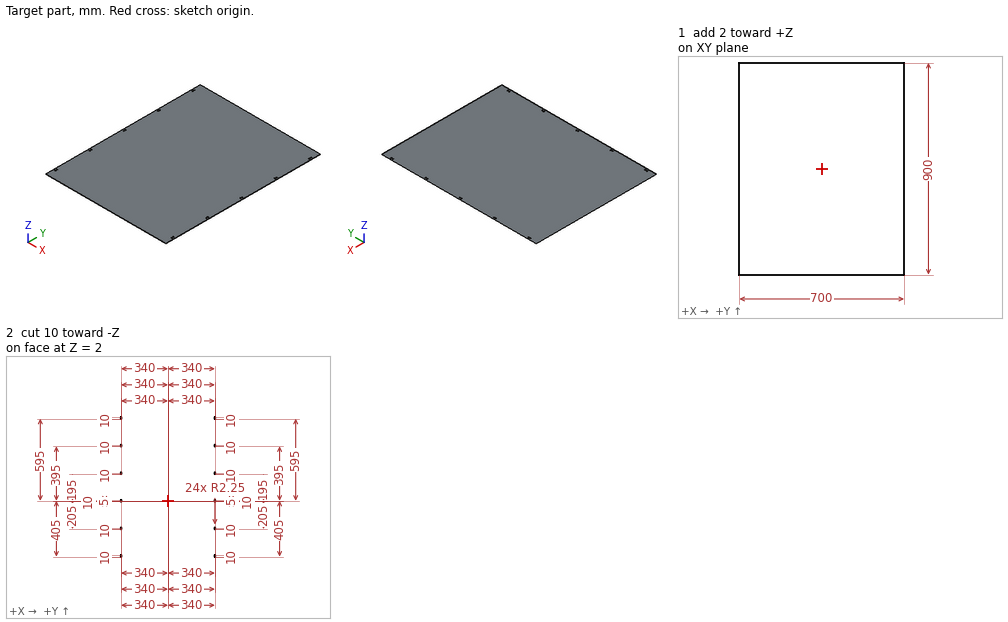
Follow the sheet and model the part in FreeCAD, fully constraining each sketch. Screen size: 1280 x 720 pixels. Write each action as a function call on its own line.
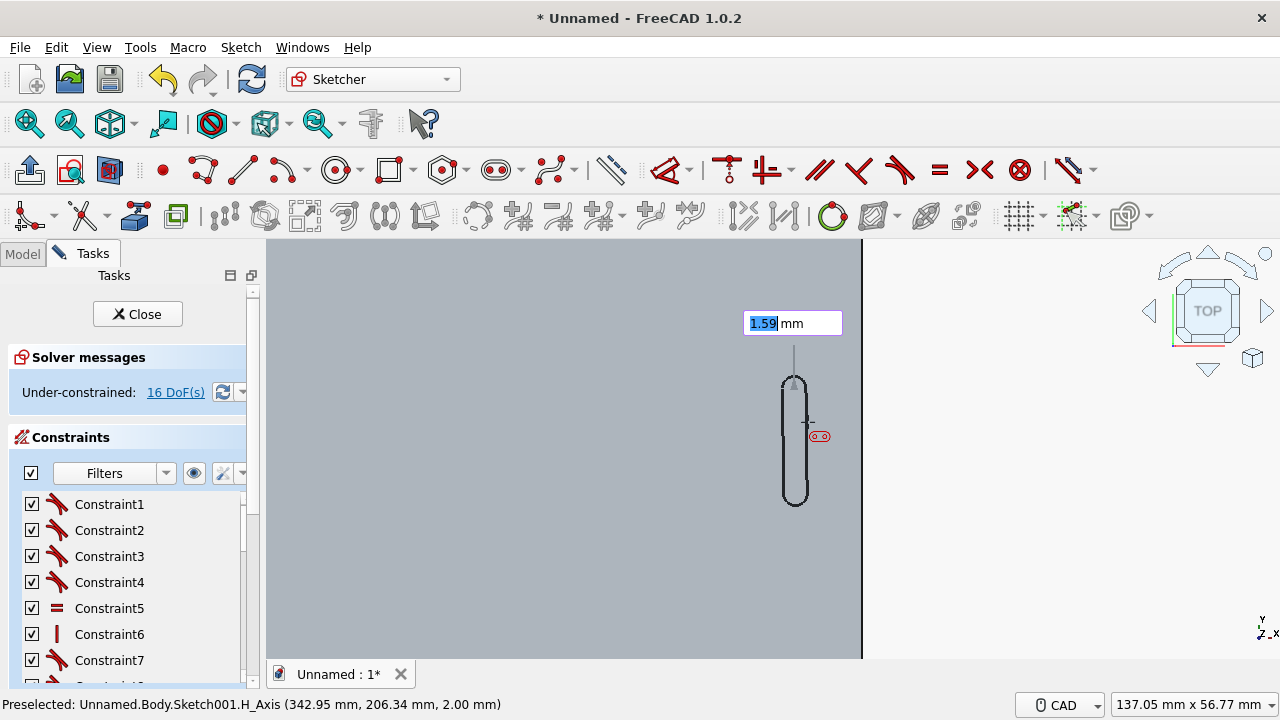
click(804, 422)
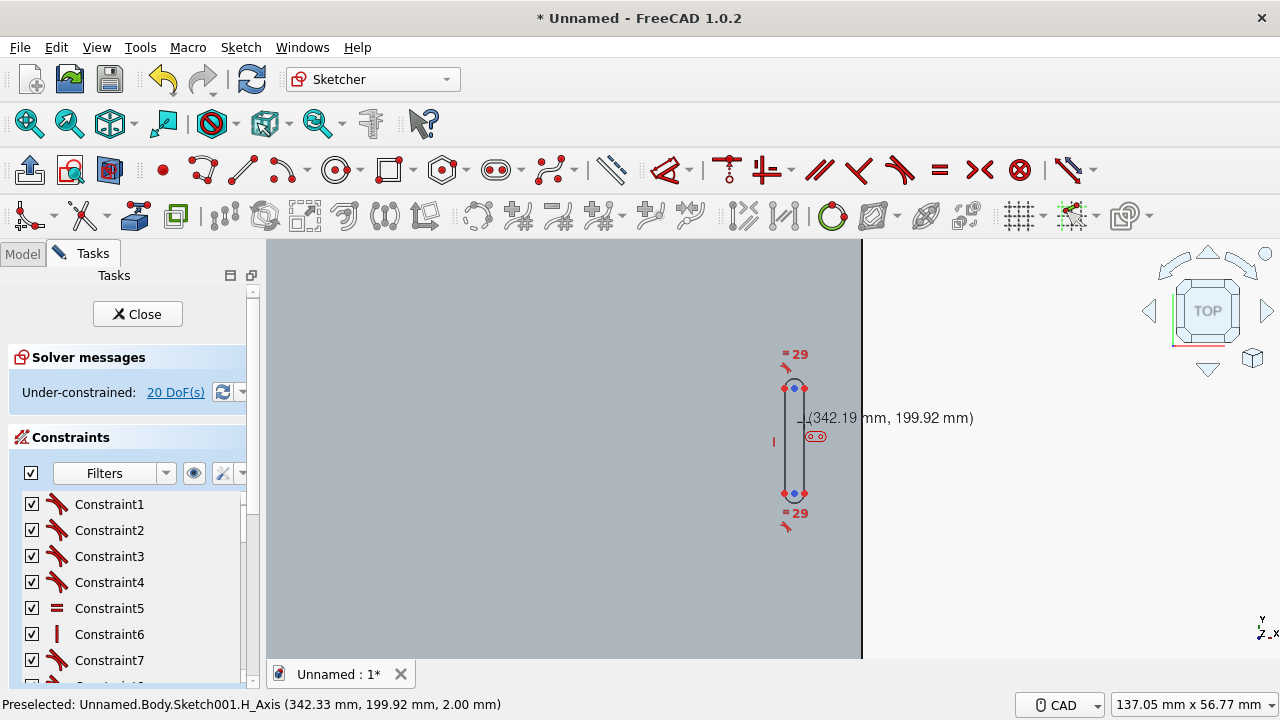
scroll(808, 419, down, 16)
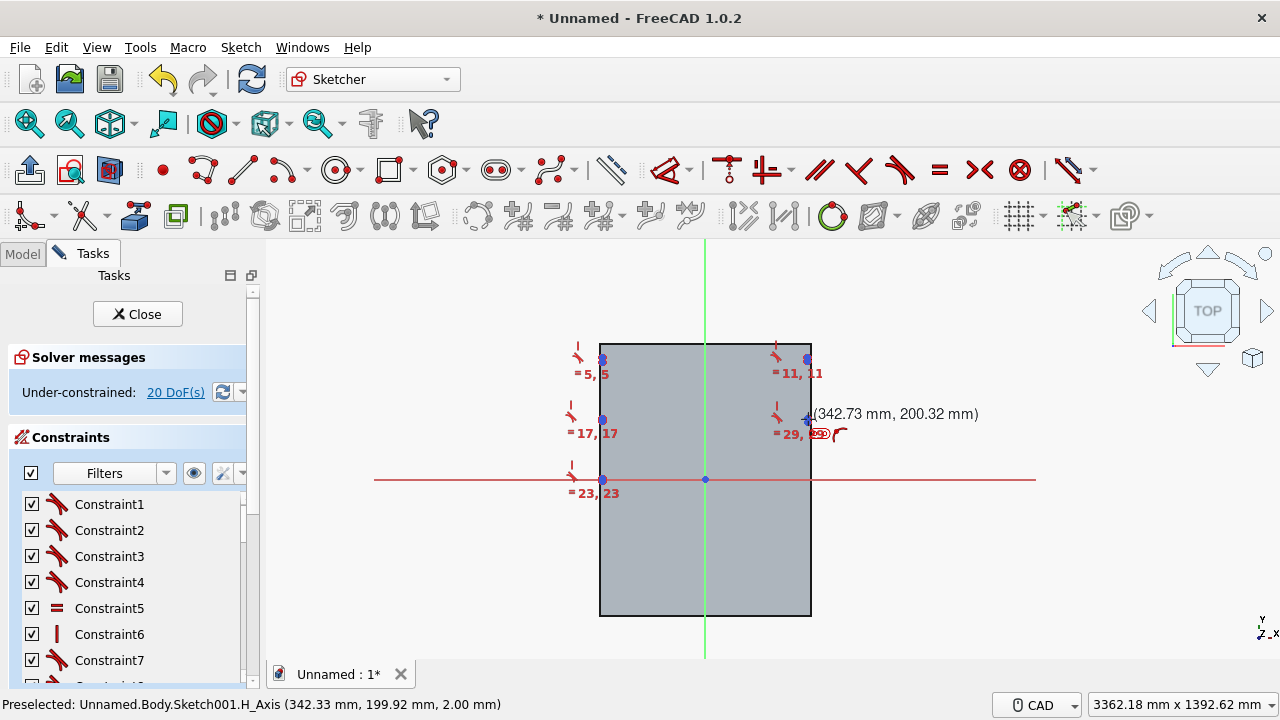
scroll(808, 481, up, 18)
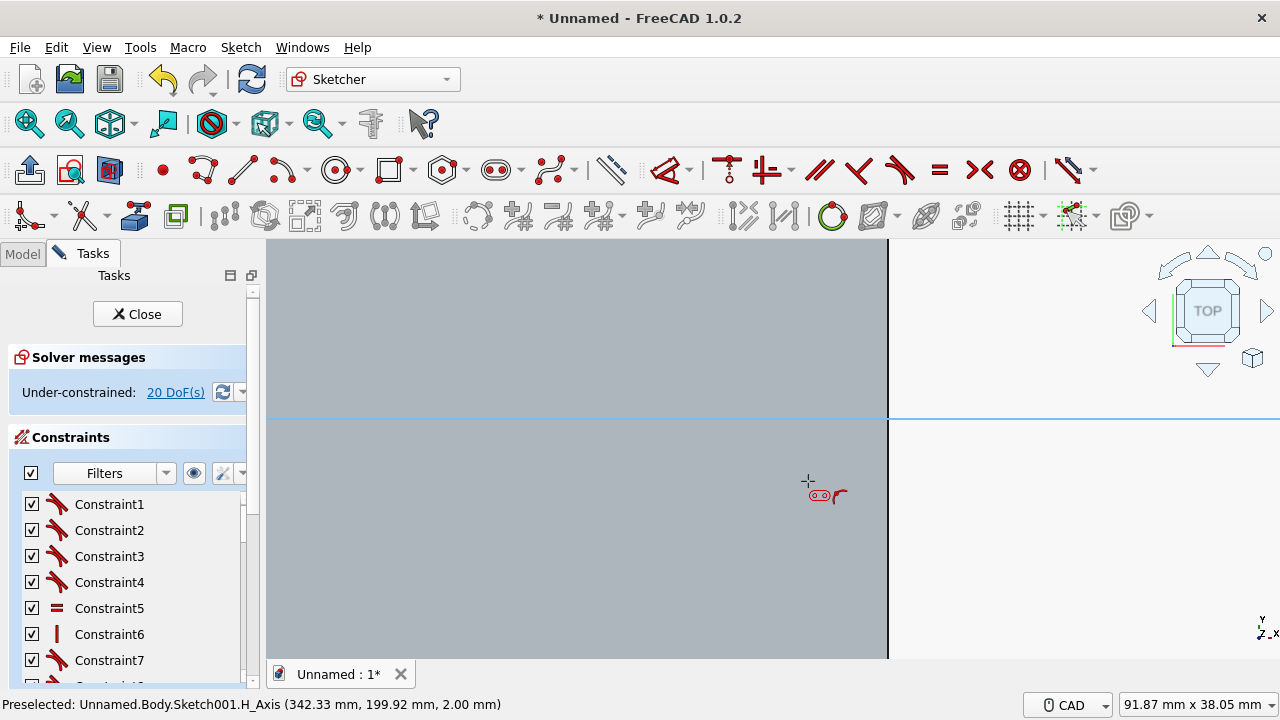
scroll(808, 481, down, 18)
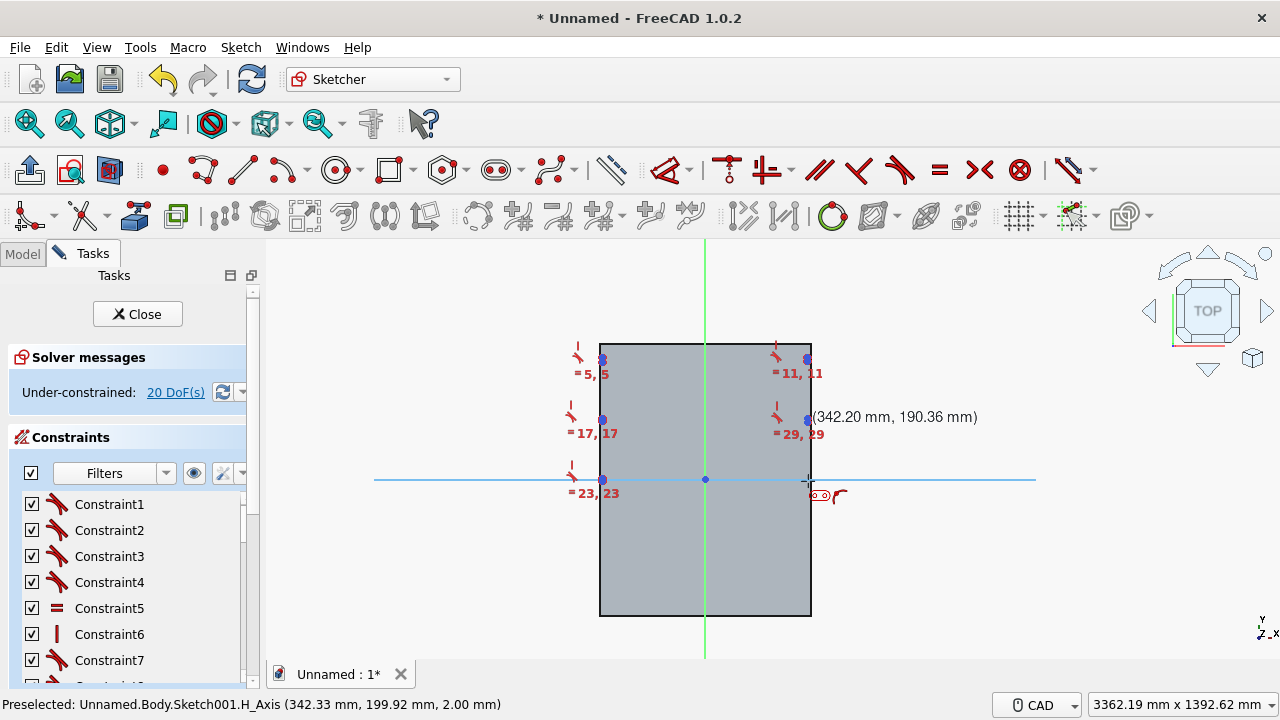
scroll(808, 481, up, 12)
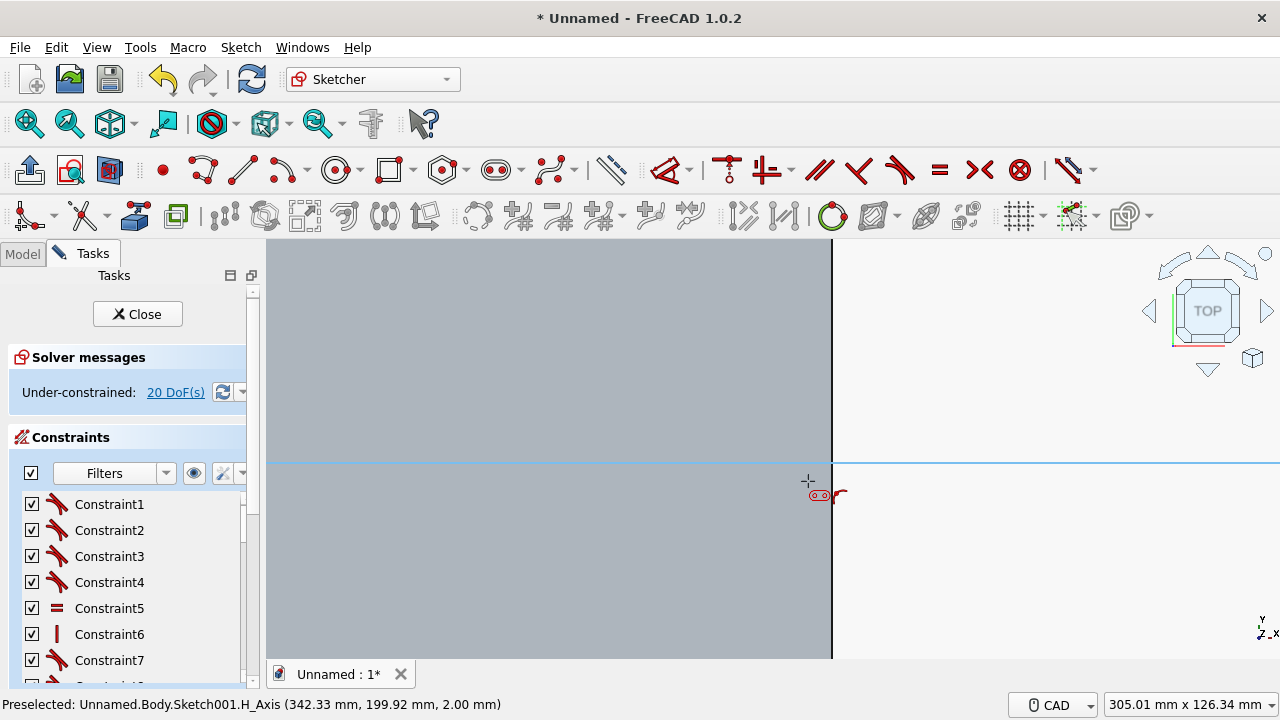
click(799, 479)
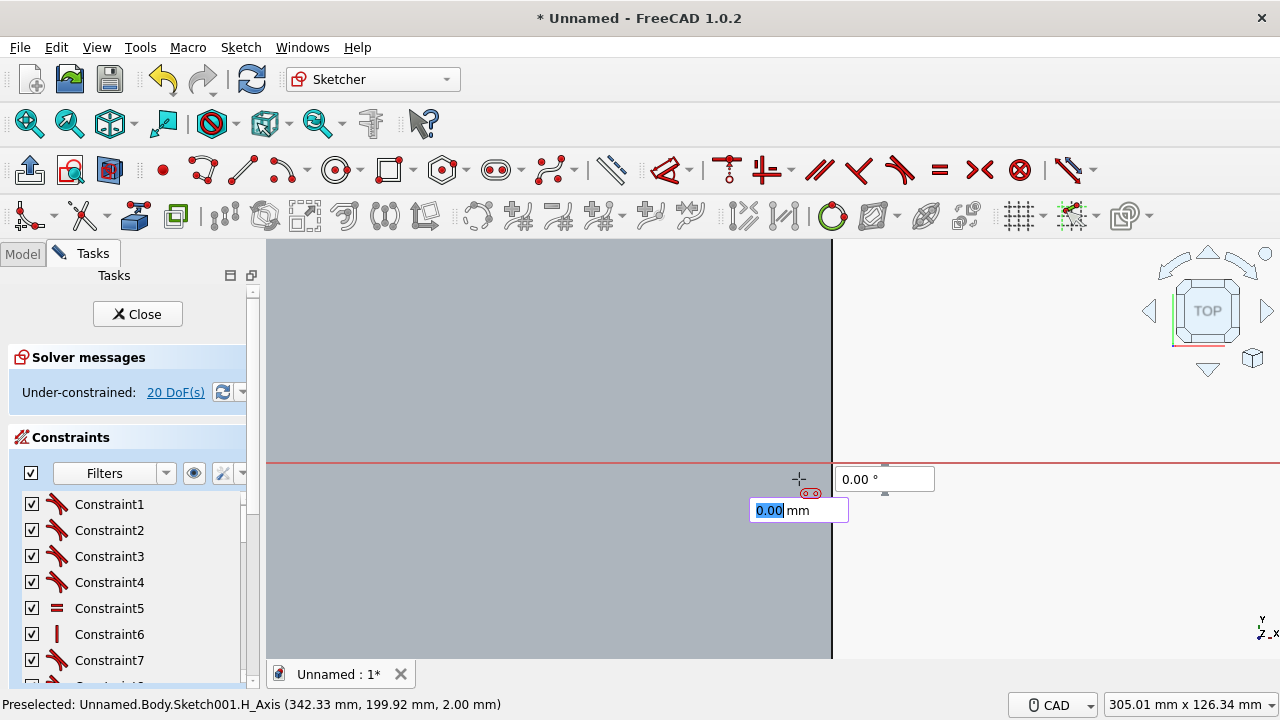
click(799, 446)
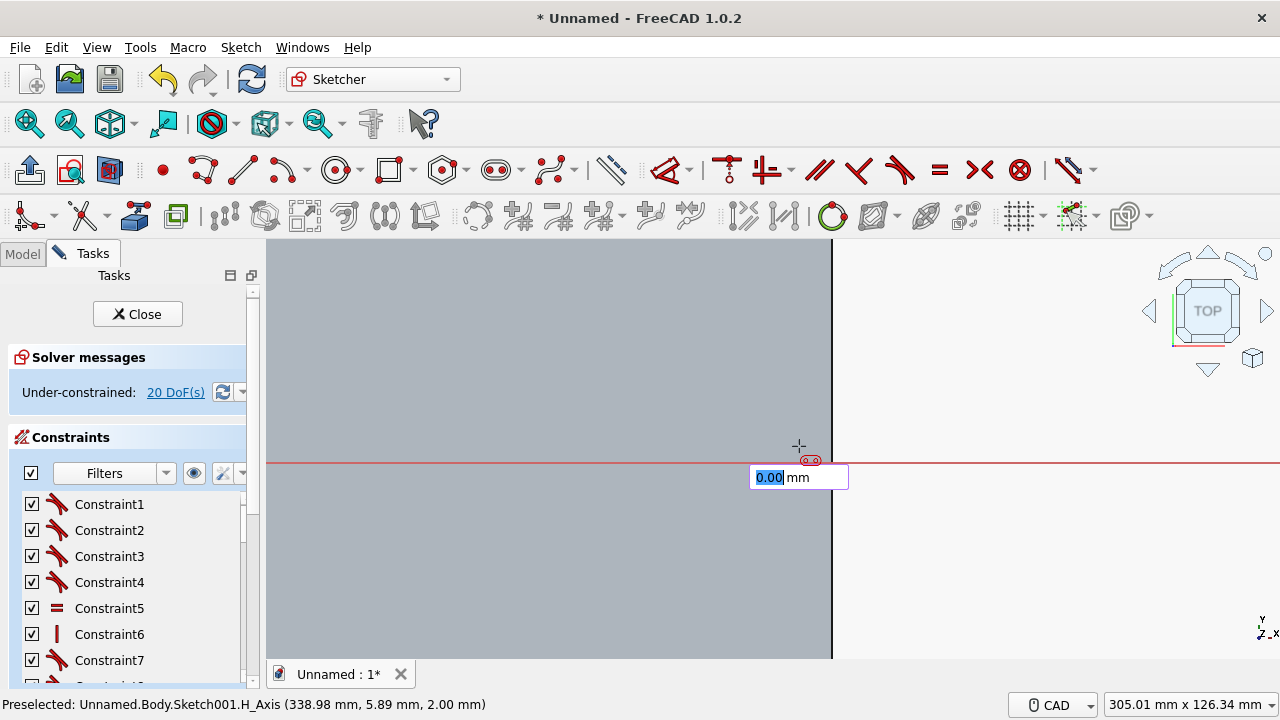
scroll(807, 468, up, 6)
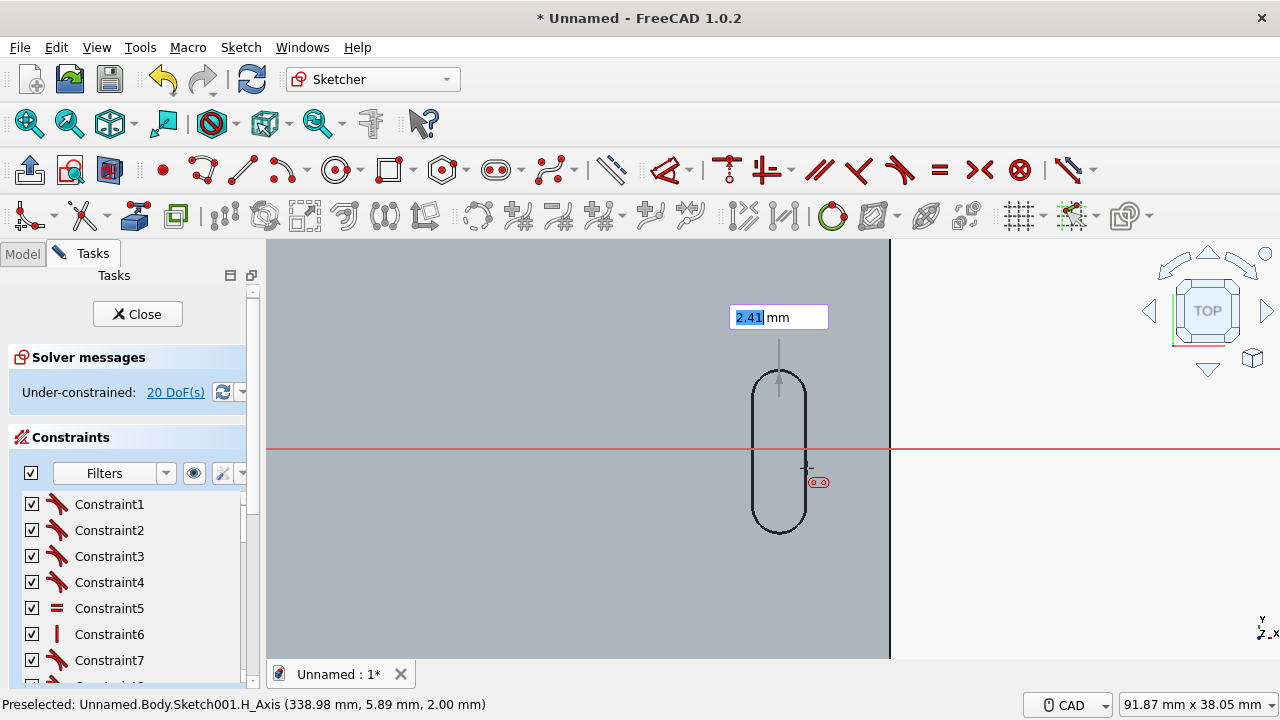
click(805, 466)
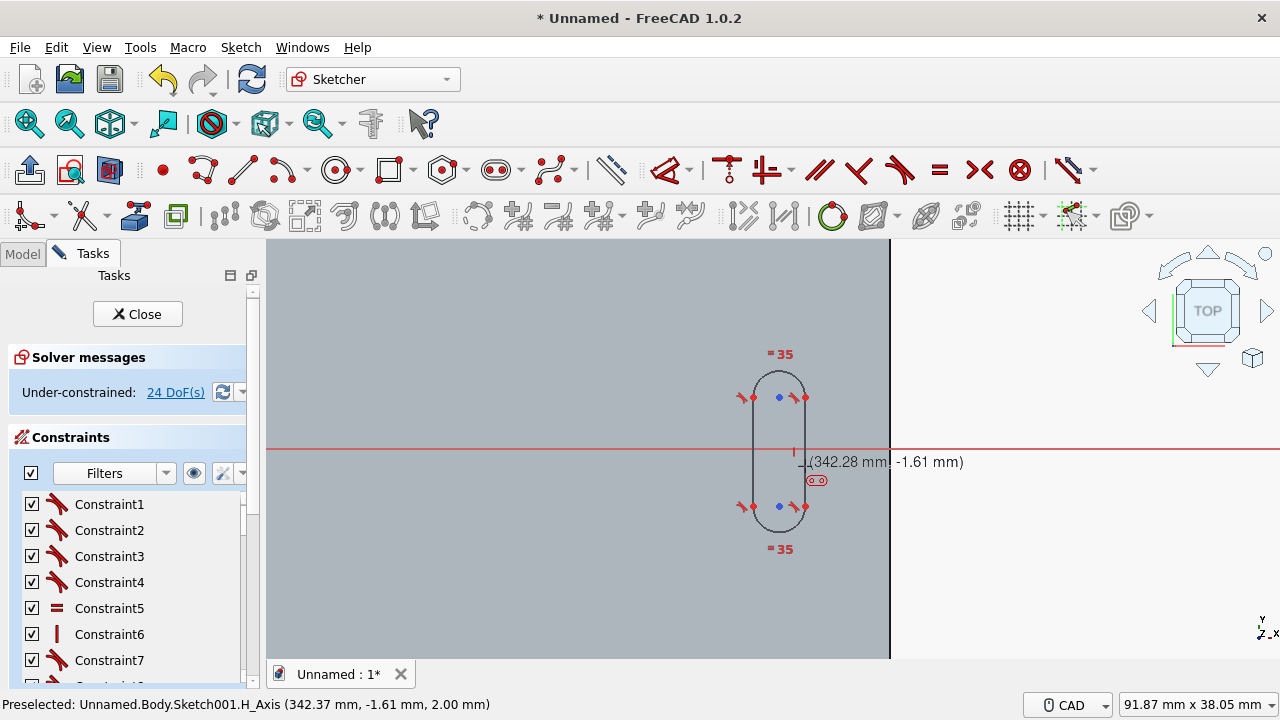
scroll(808, 480, down, 18)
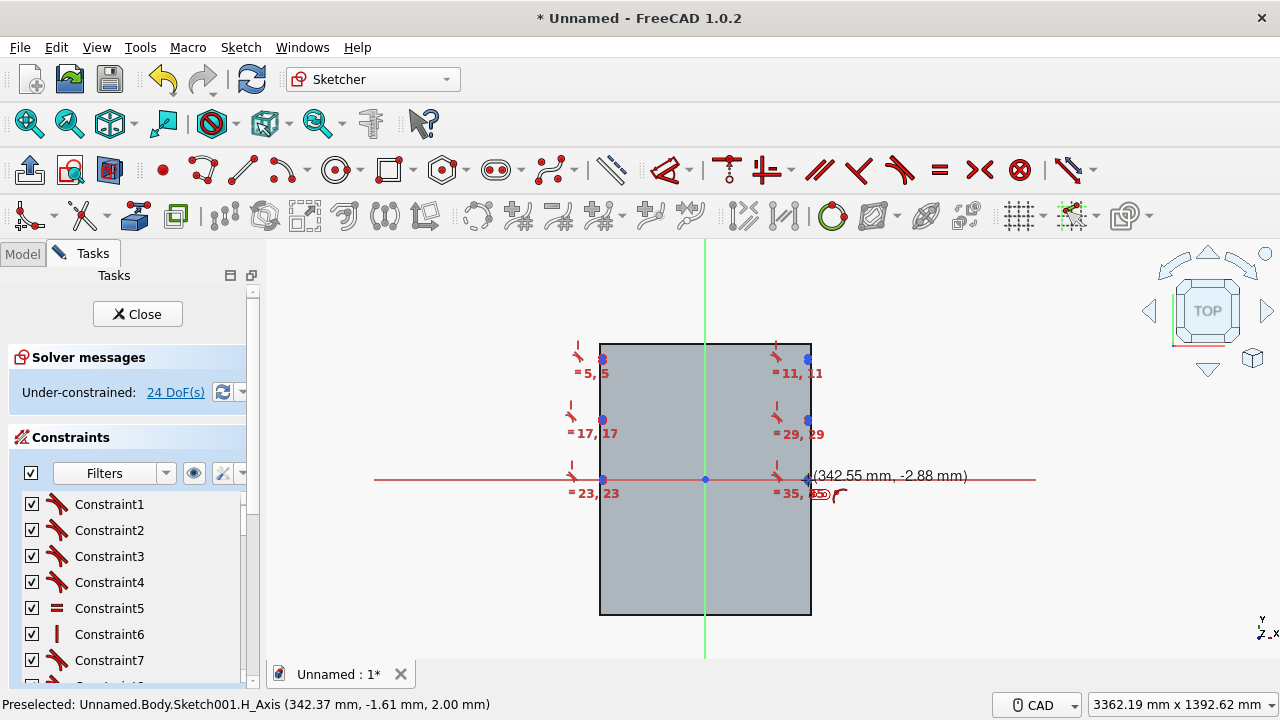
scroll(603, 300, up, 18)